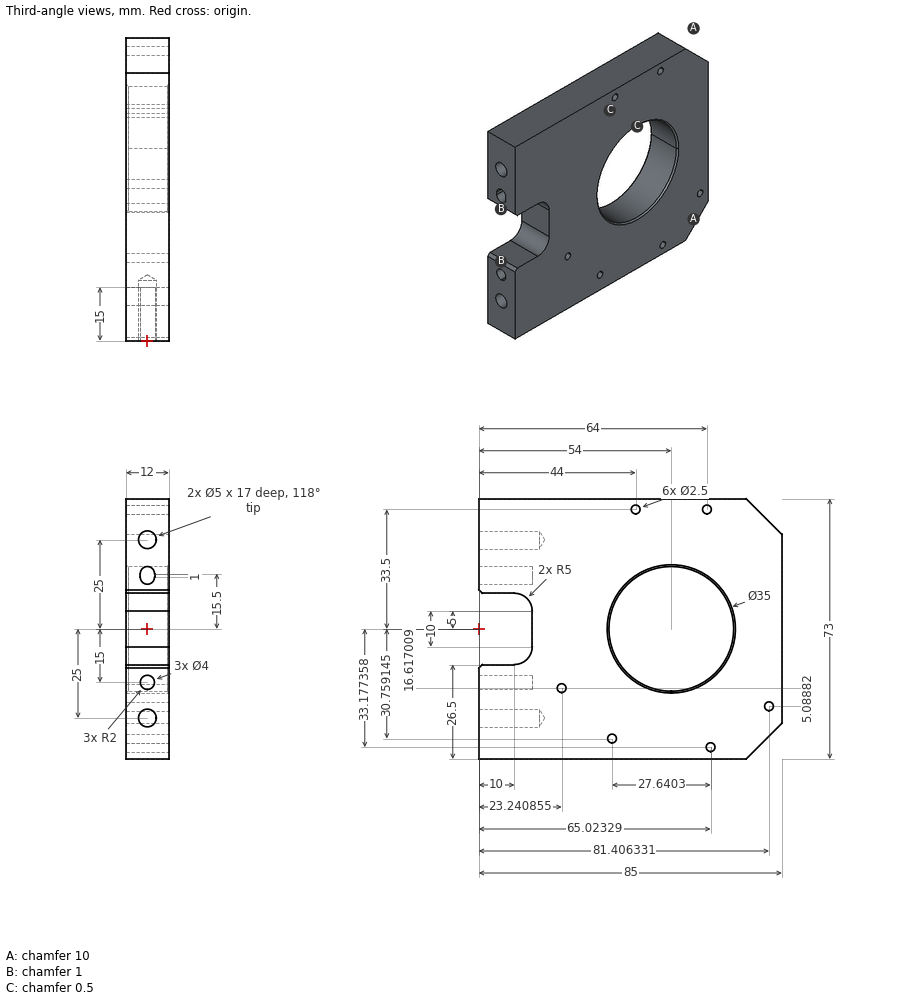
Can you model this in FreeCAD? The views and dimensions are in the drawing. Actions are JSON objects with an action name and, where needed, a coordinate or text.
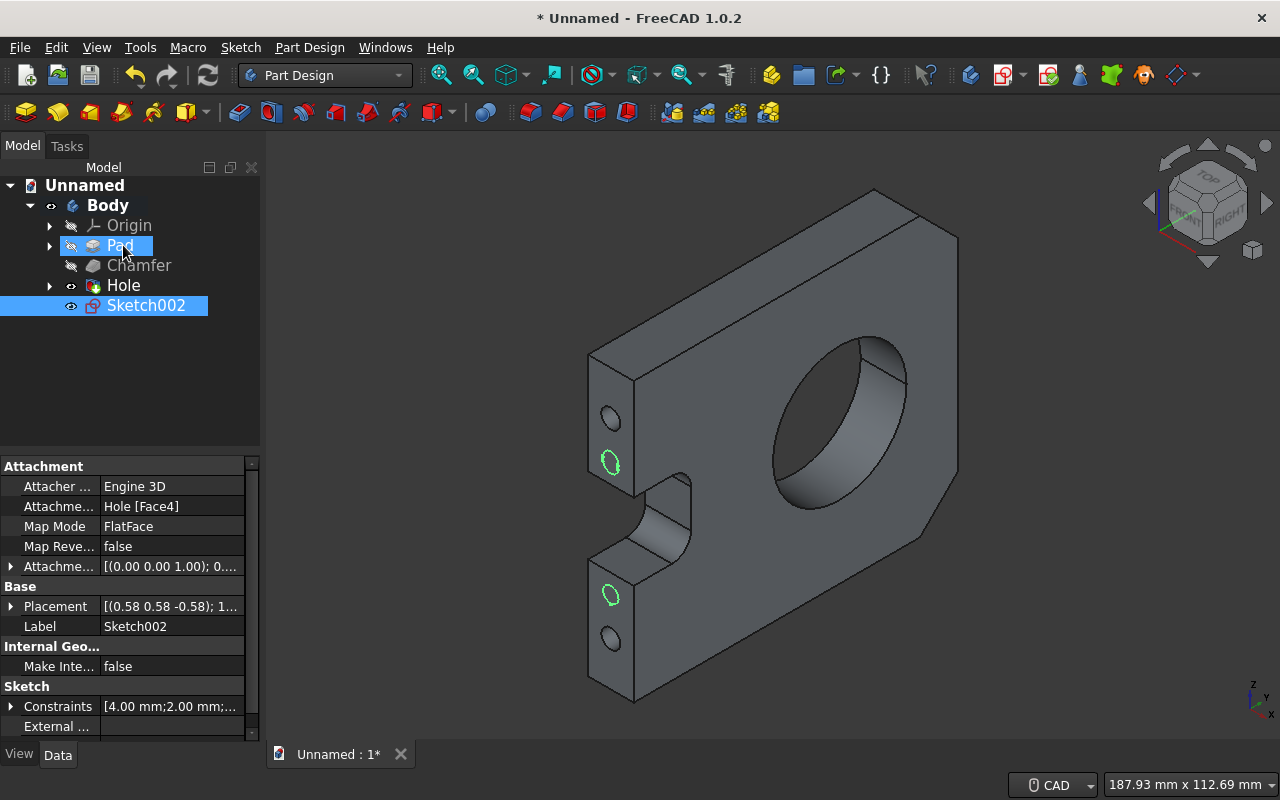
{"action": "left_click", "coordinate": [240, 112]}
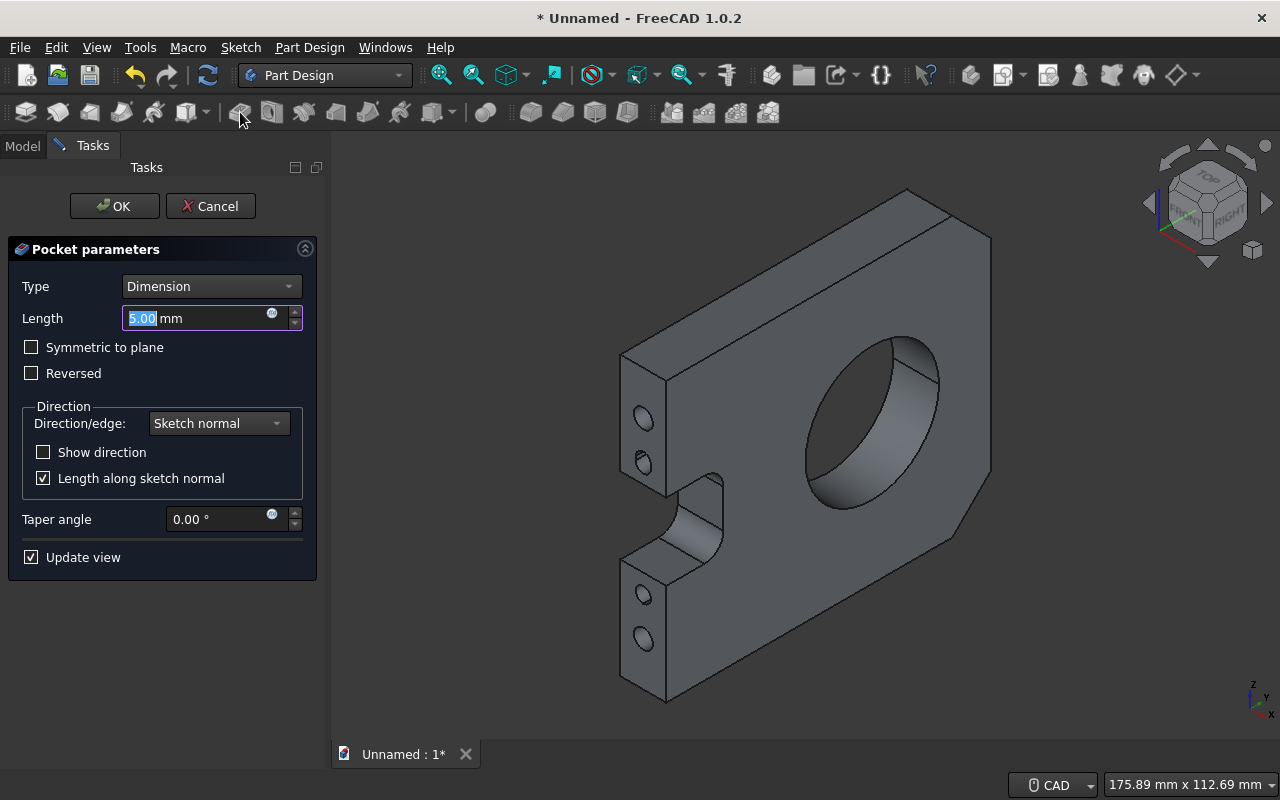
{"action": "type", "text": "15"}
{"action": "key", "text": "Tab"}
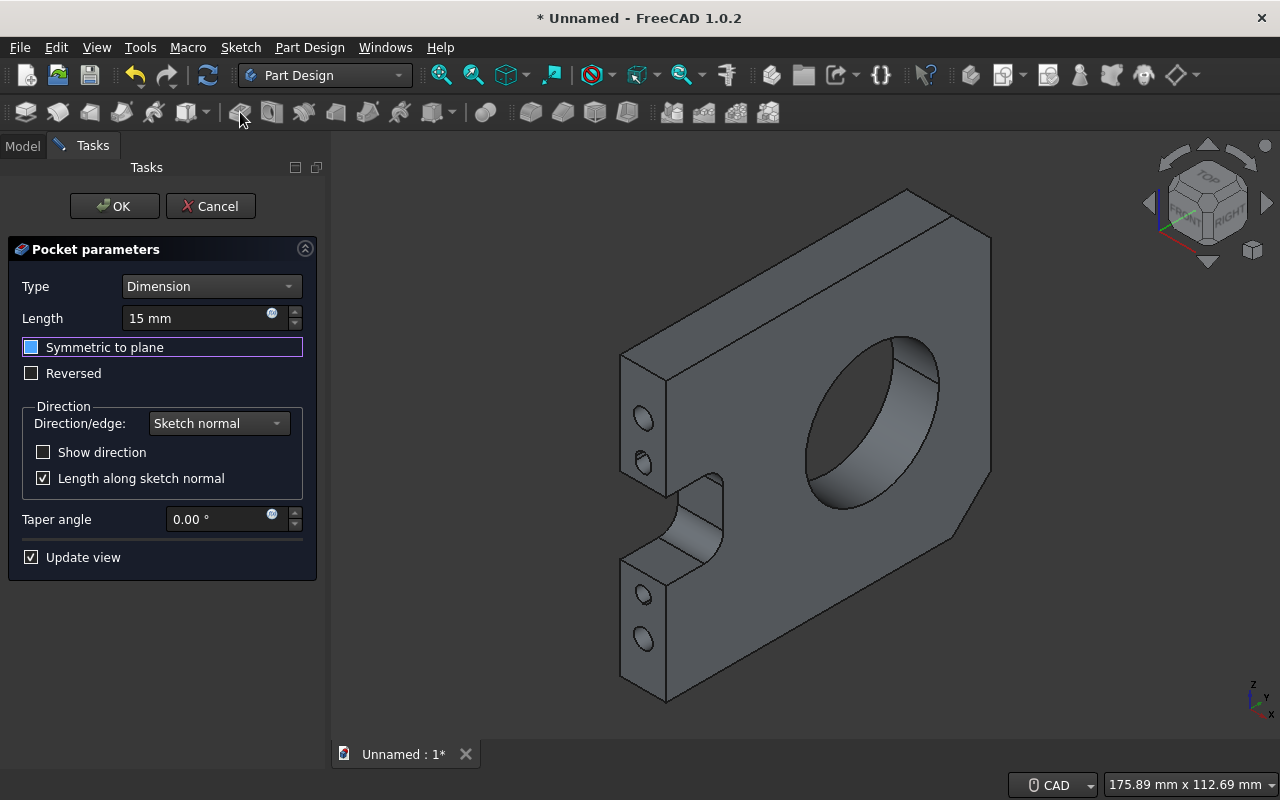
{"action": "left_click", "coordinate": [115, 206]}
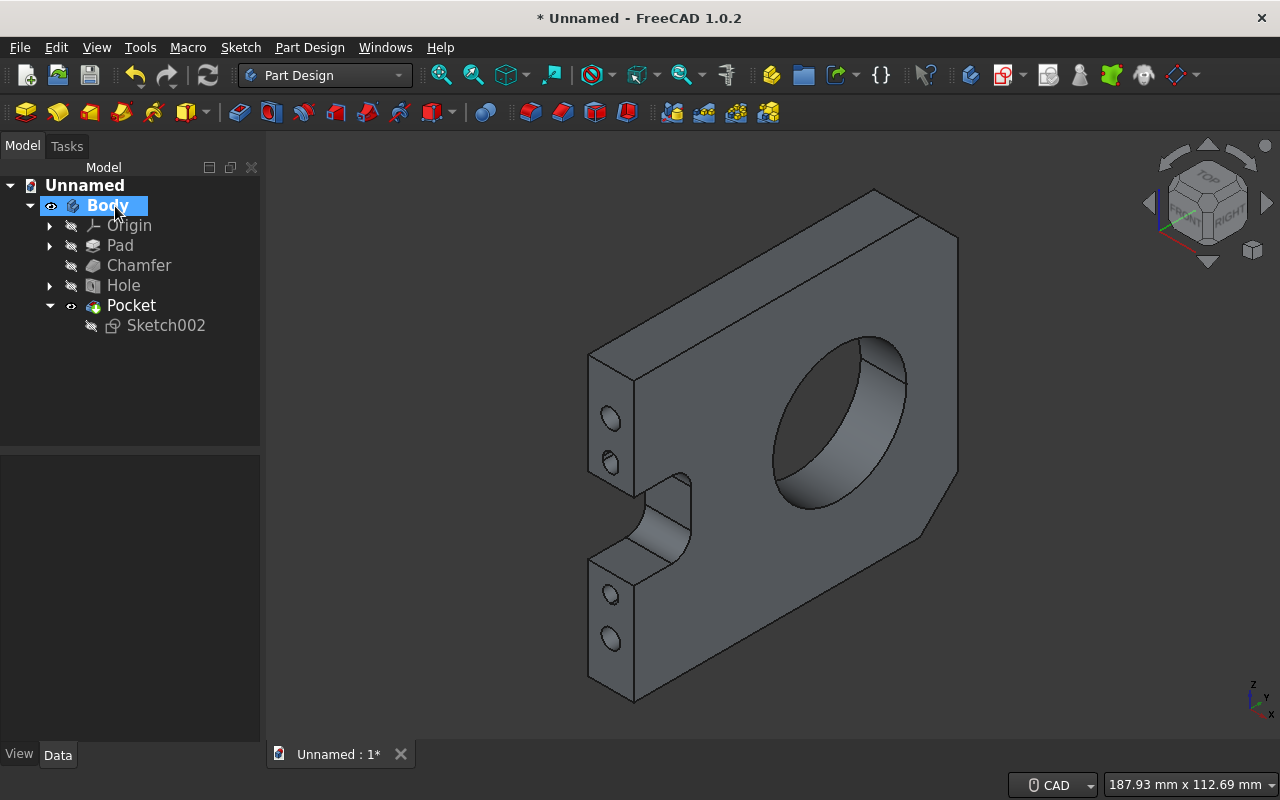
{"action": "left_click", "coordinate": [611, 572]}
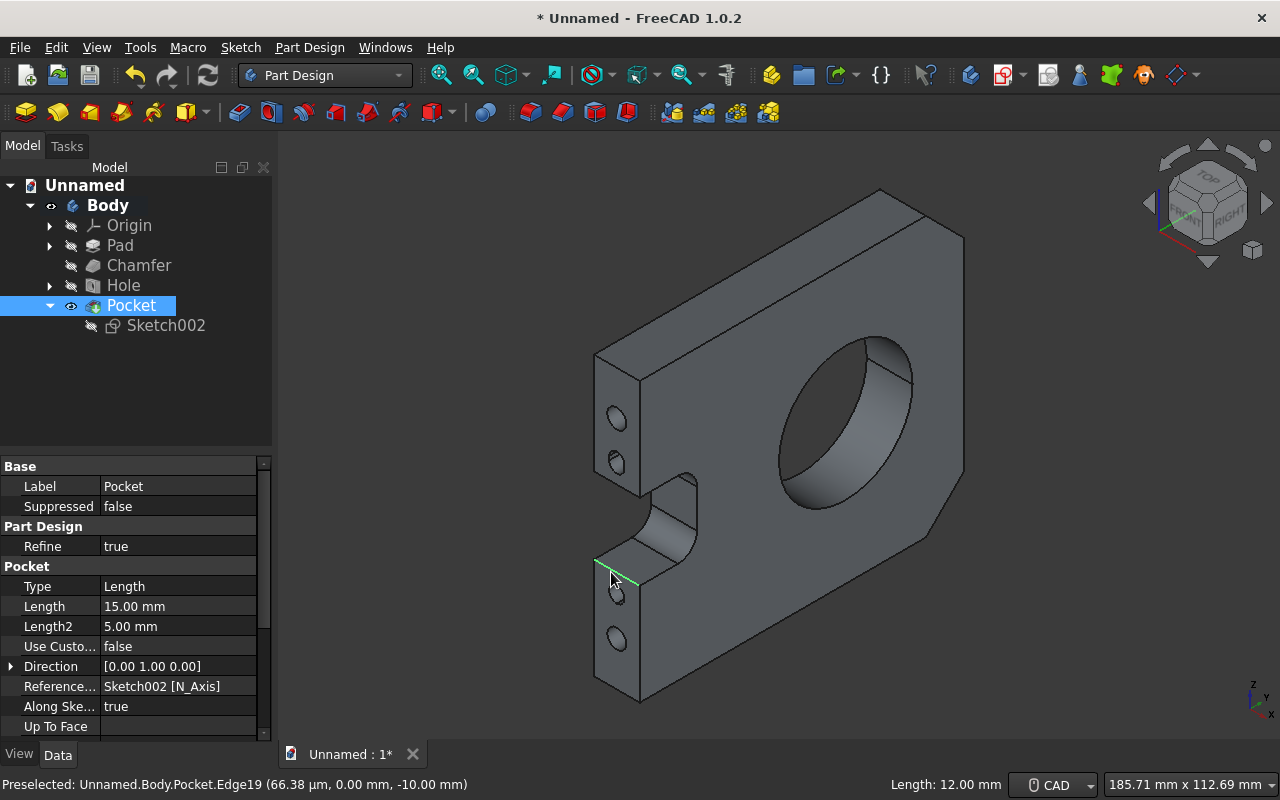
{"action": "key", "text": "2"}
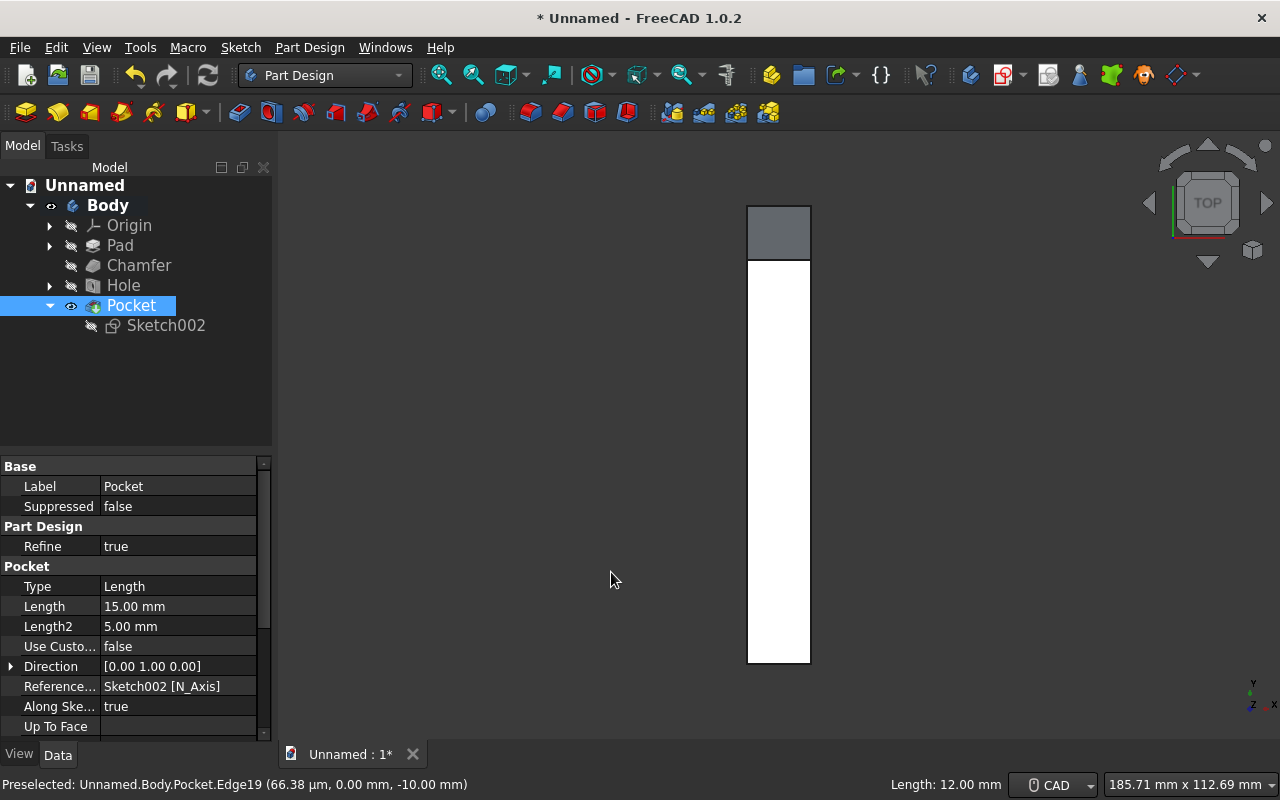
{"action": "key", "text": "0"}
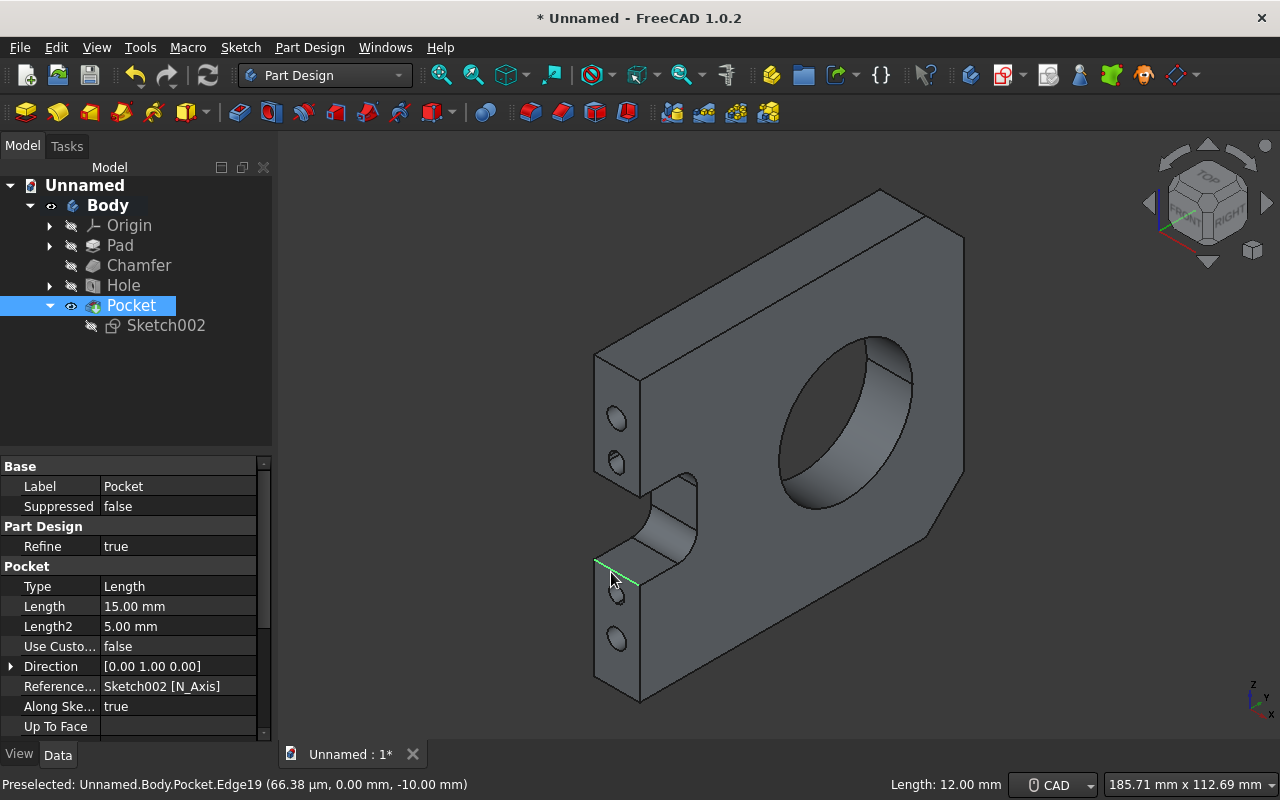
{"action": "key", "text": "1"}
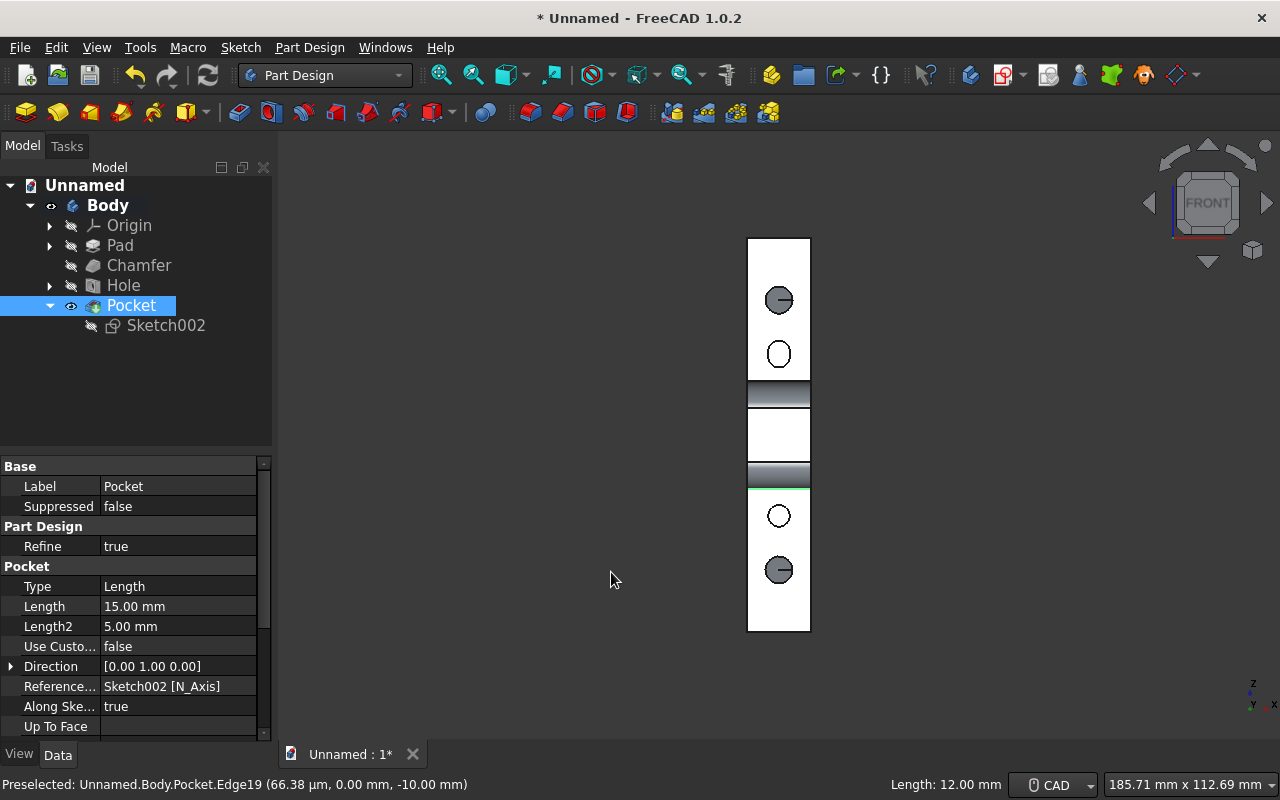
{"action": "left_click", "coordinate": [779, 380], "text": "ctrl"}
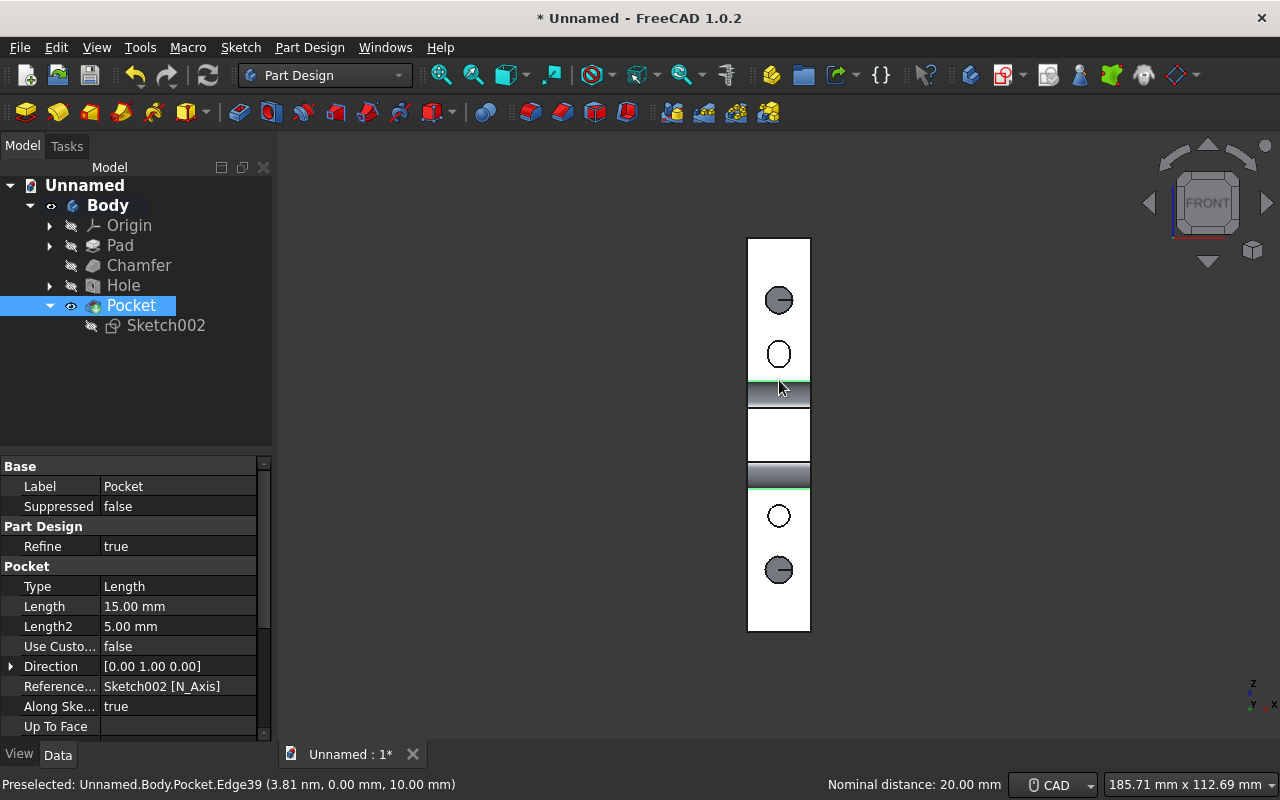
{"action": "left_click", "coordinate": [564, 112]}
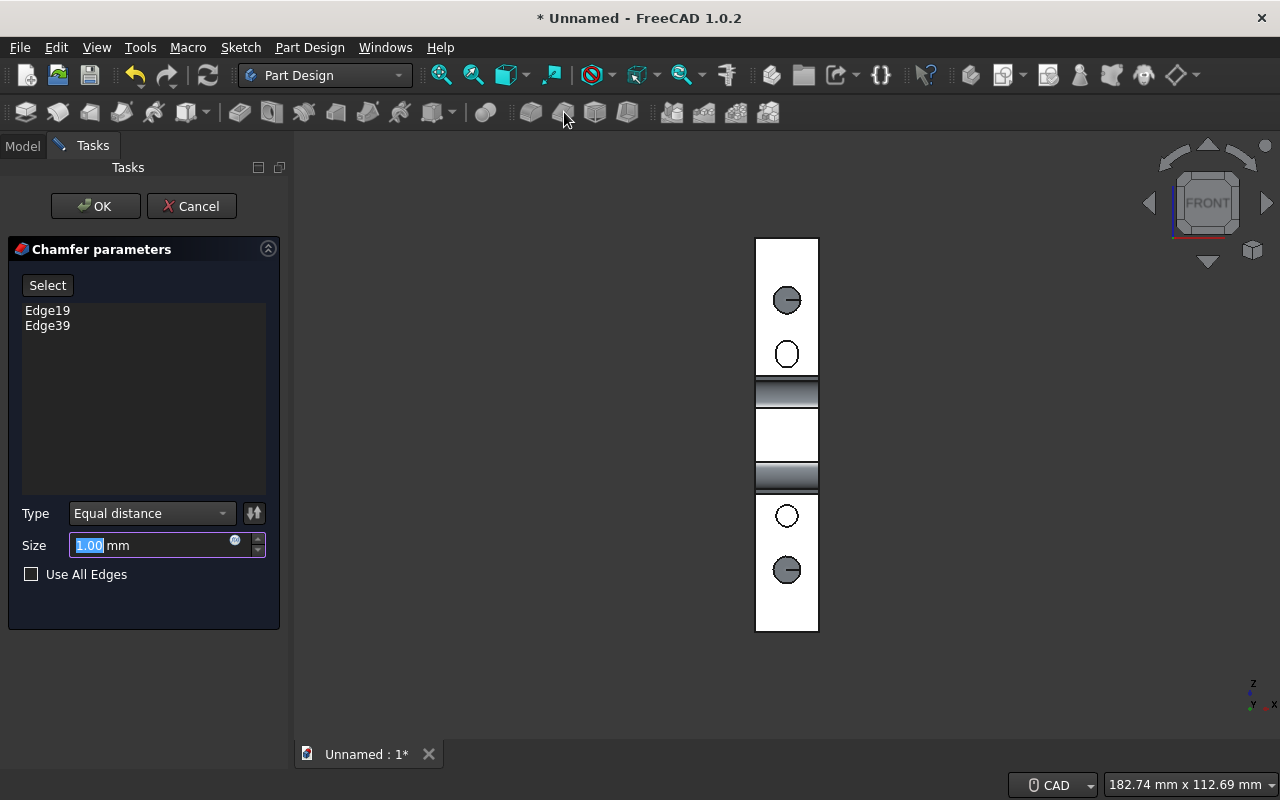
{"action": "type", "text": "1"}
{"action": "key", "text": "Tab"}